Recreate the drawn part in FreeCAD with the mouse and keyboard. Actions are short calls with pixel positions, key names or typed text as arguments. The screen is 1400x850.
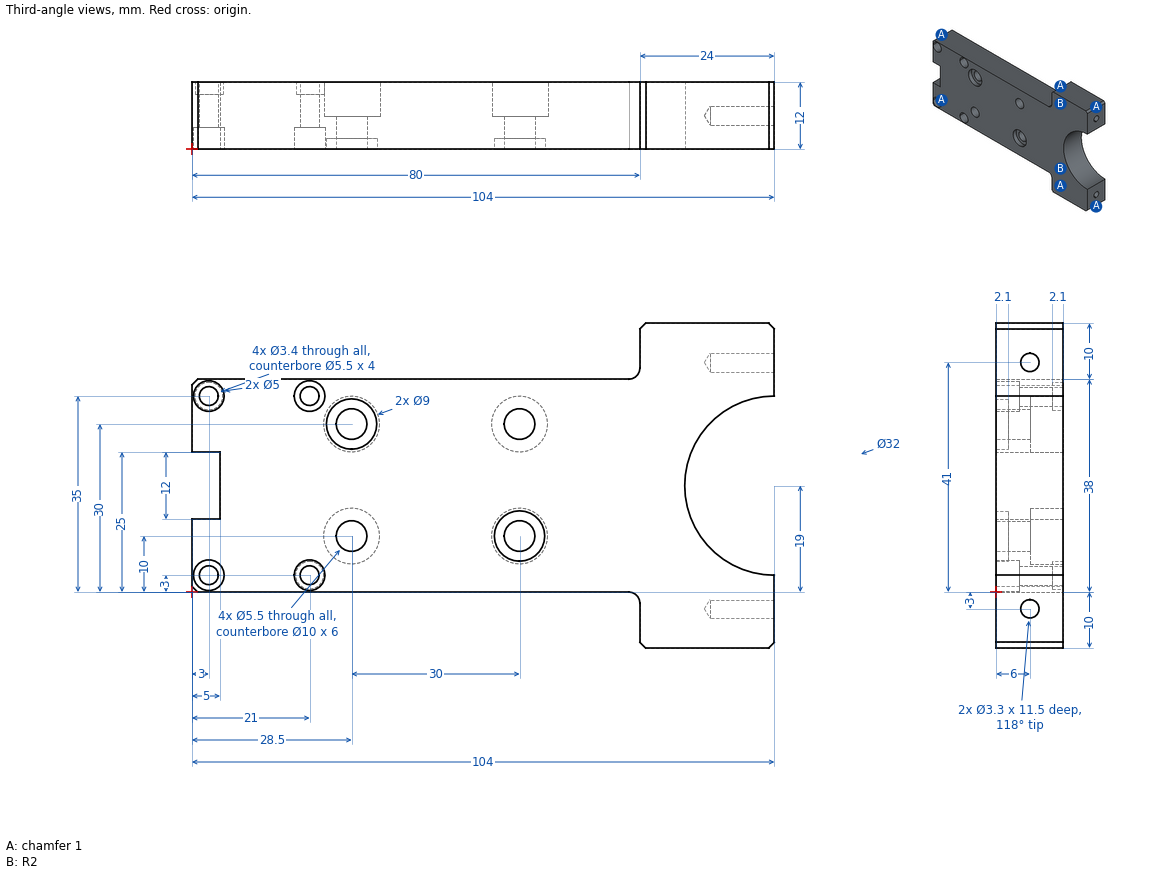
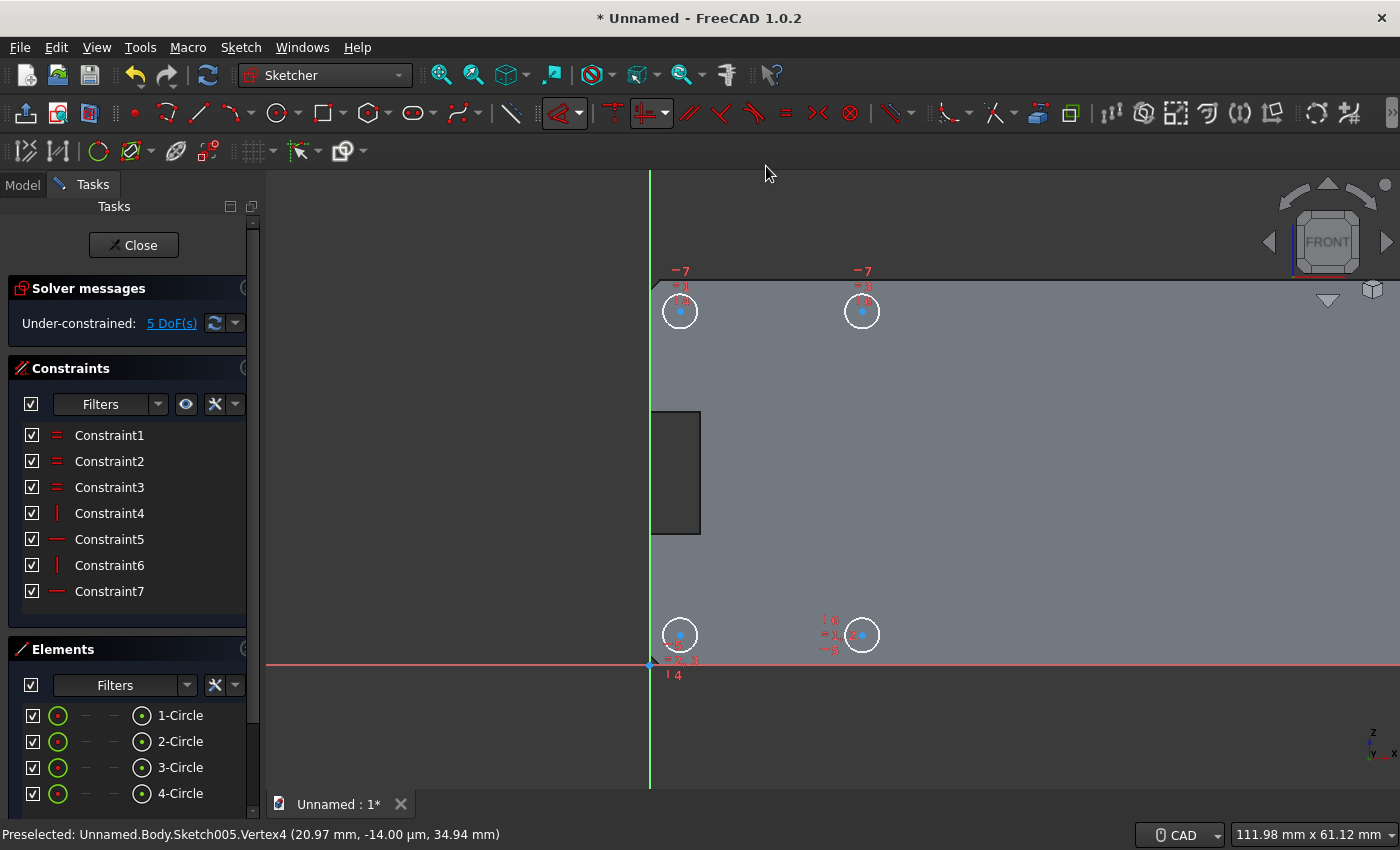
click(692, 299)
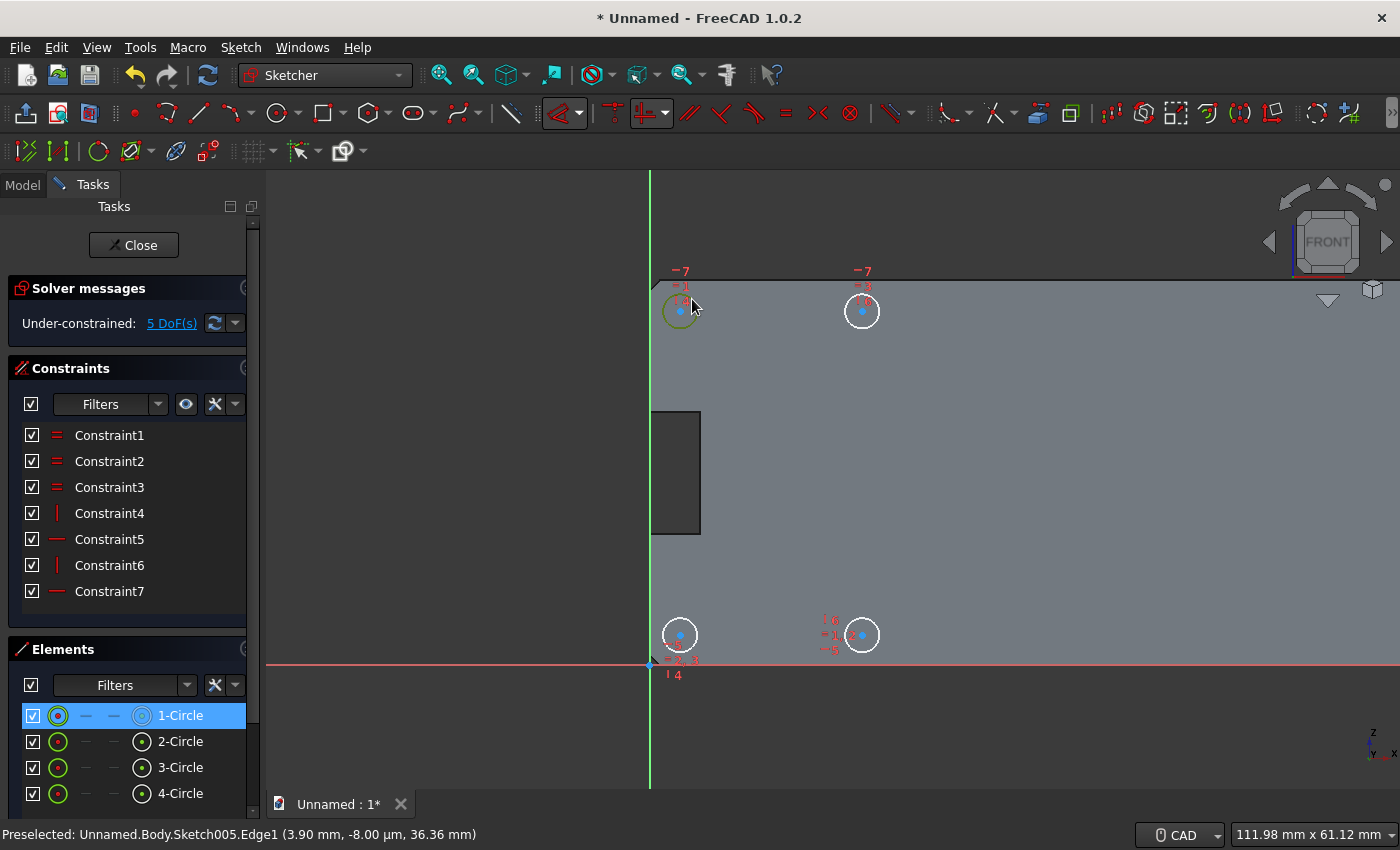
key(k)
key(o)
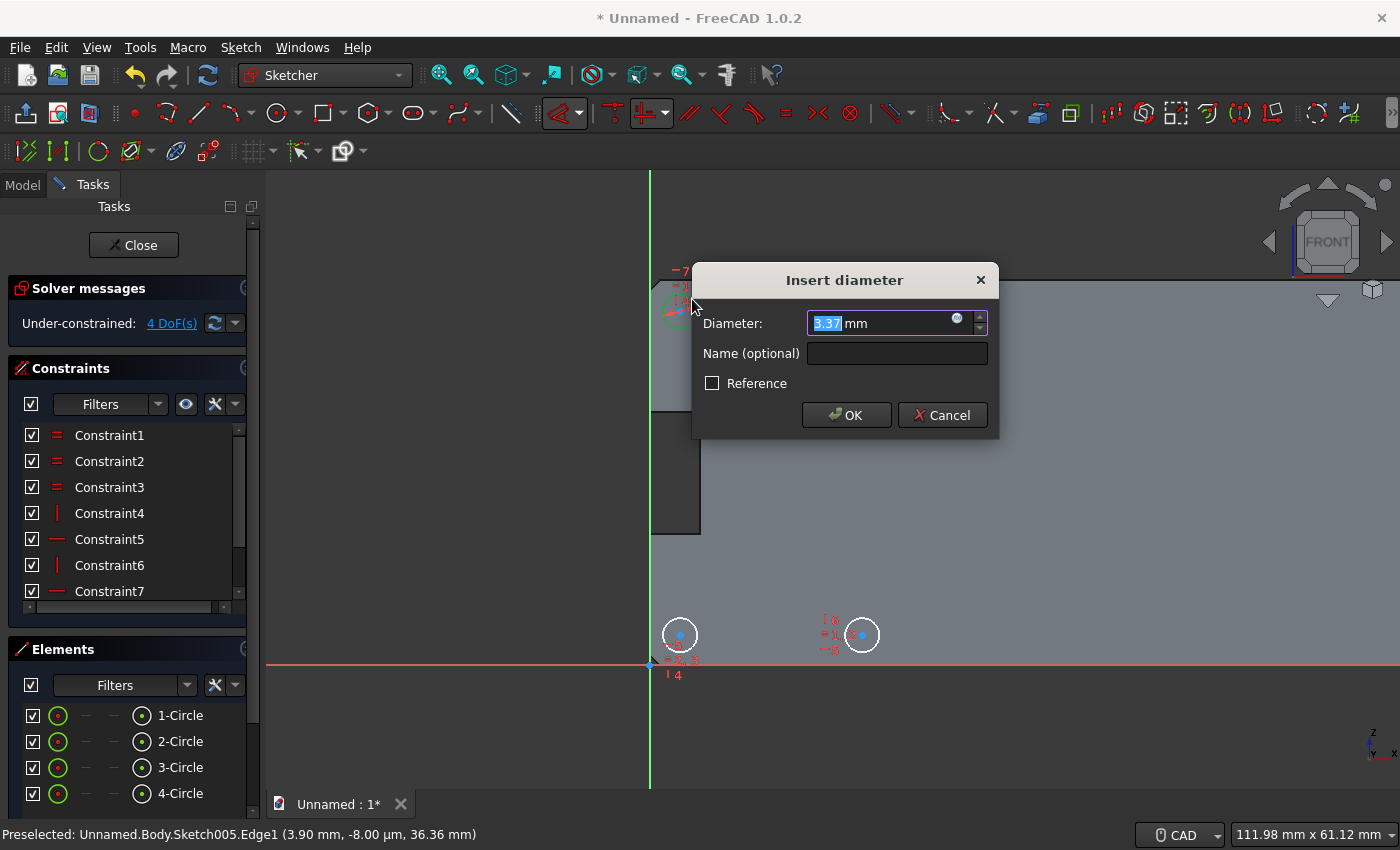
text(3.4)
key(Return)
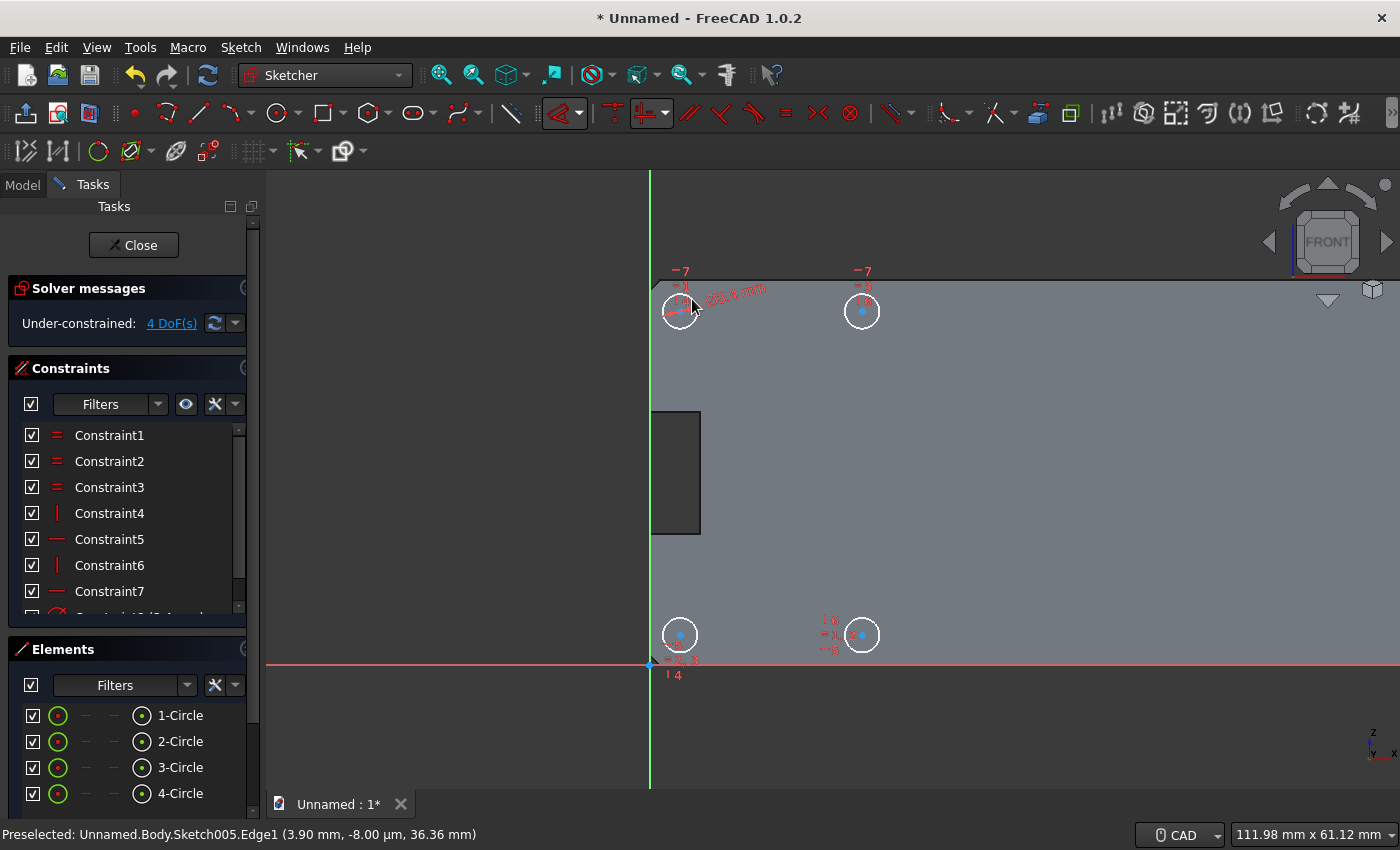
scroll(680, 311, up, 2)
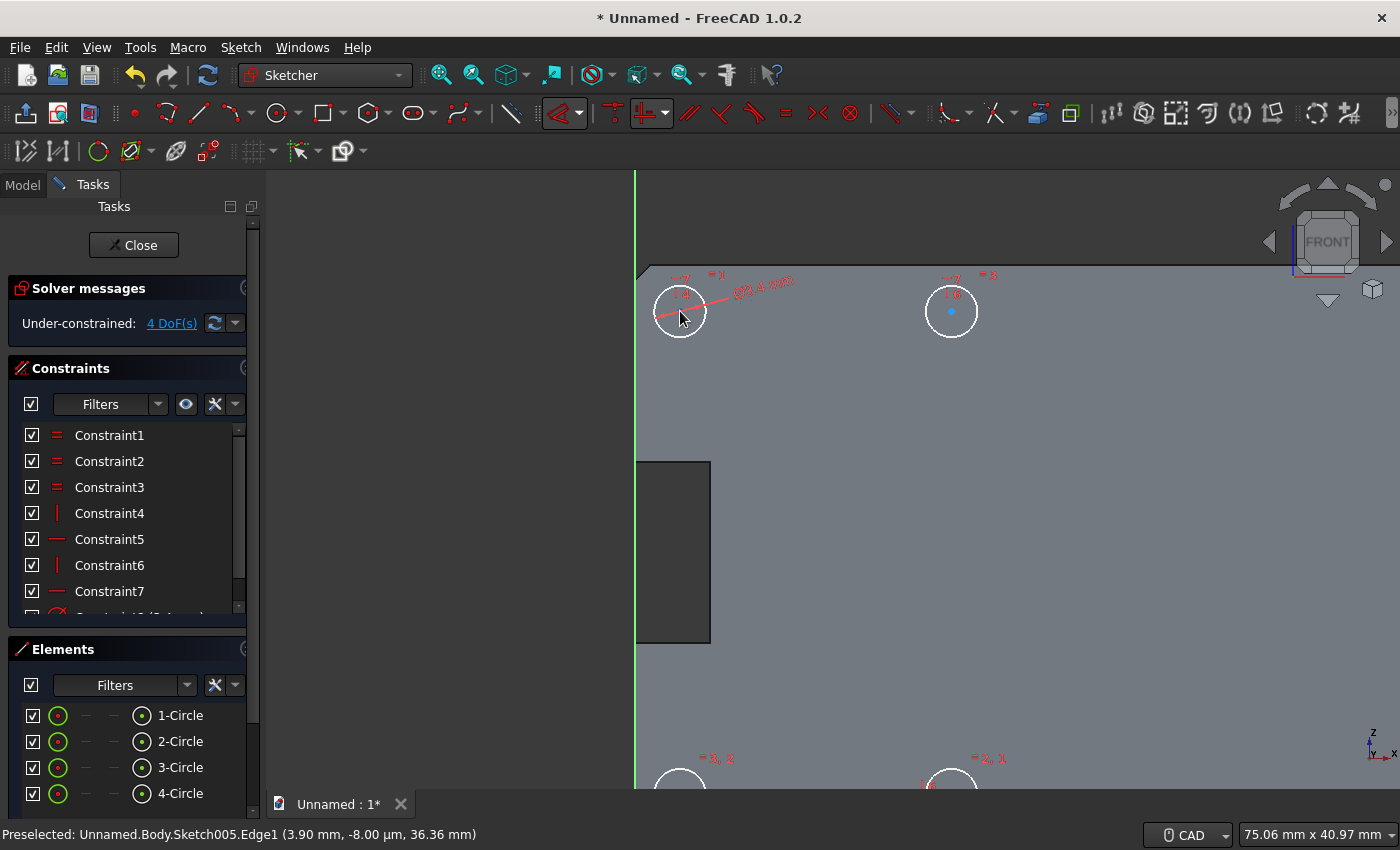
click(680, 311)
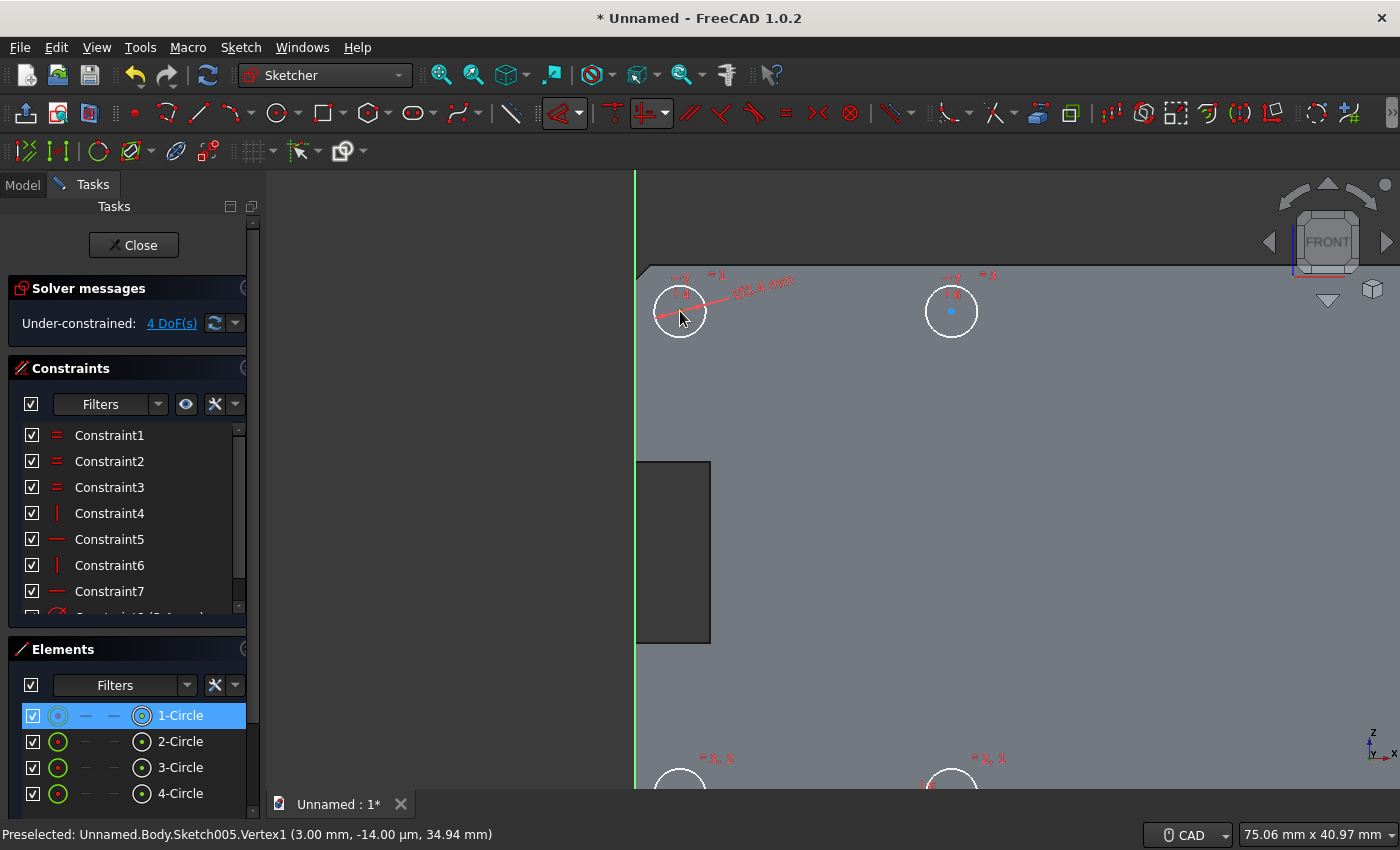
key(l)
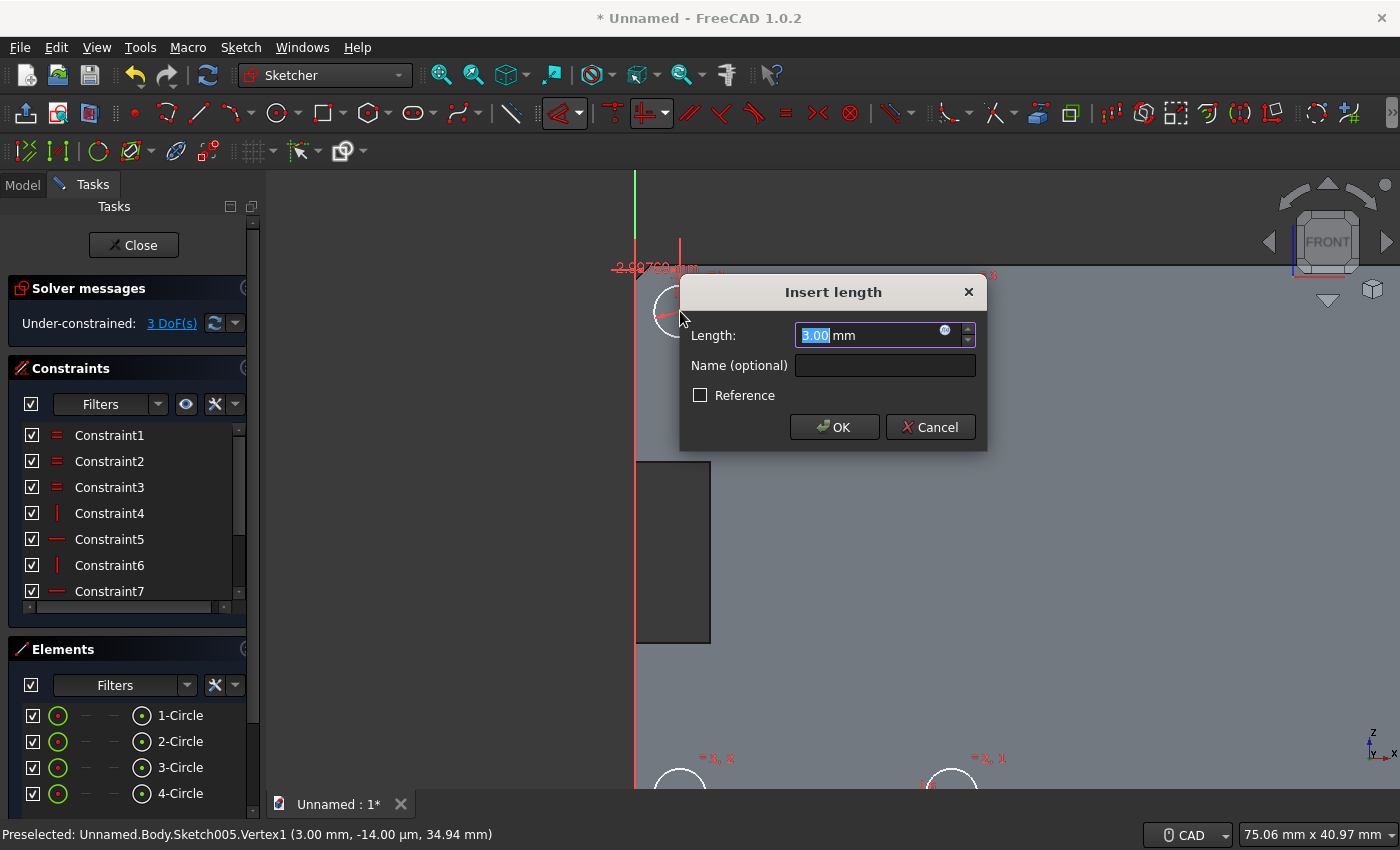
text(3)
key(Return)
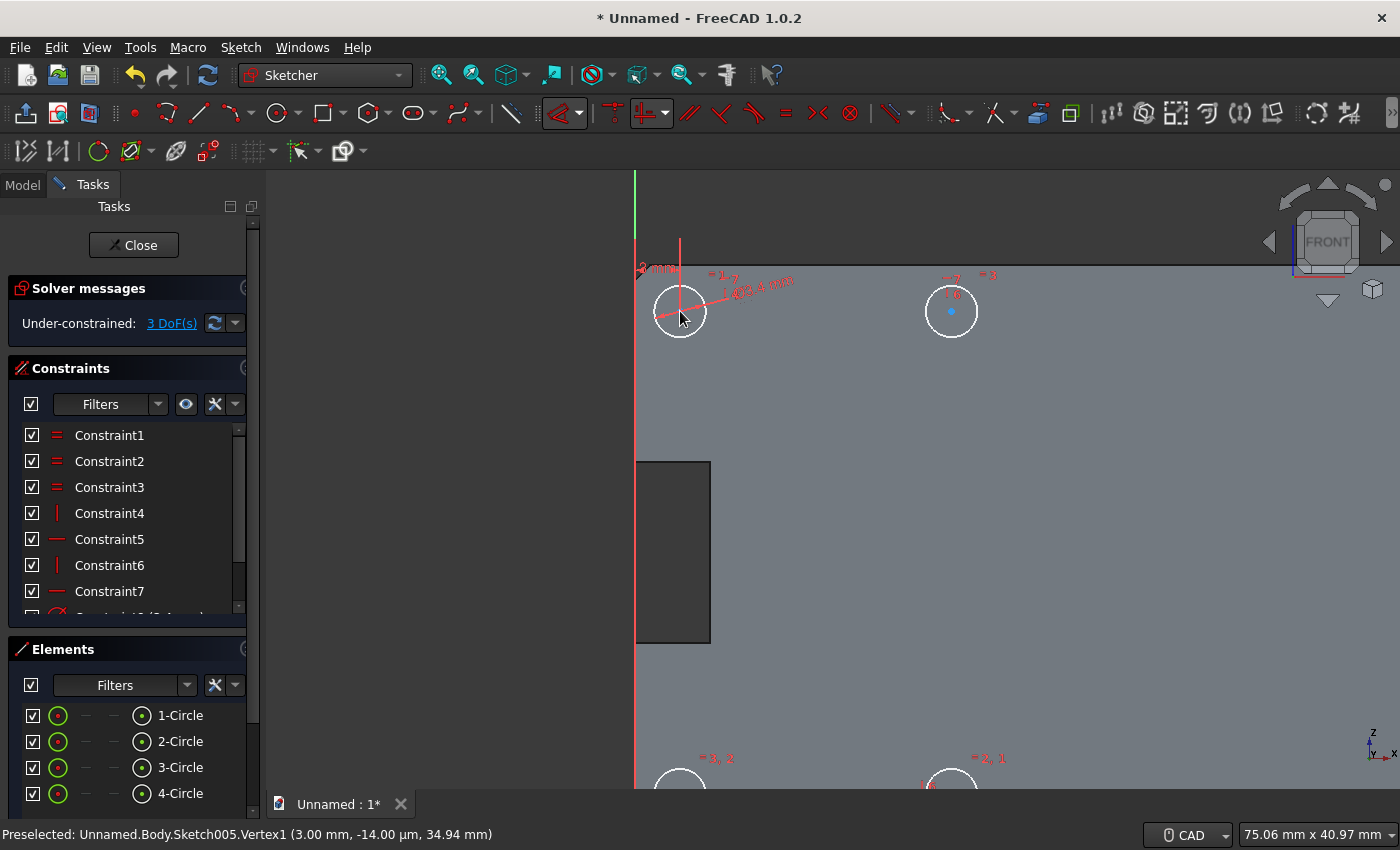
scroll(680, 311, down, 2)